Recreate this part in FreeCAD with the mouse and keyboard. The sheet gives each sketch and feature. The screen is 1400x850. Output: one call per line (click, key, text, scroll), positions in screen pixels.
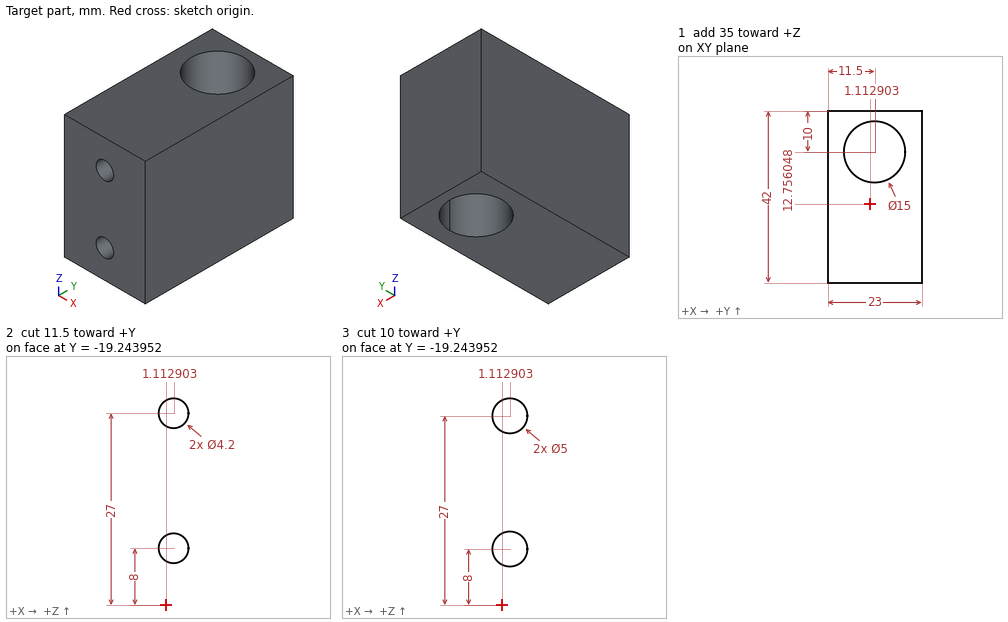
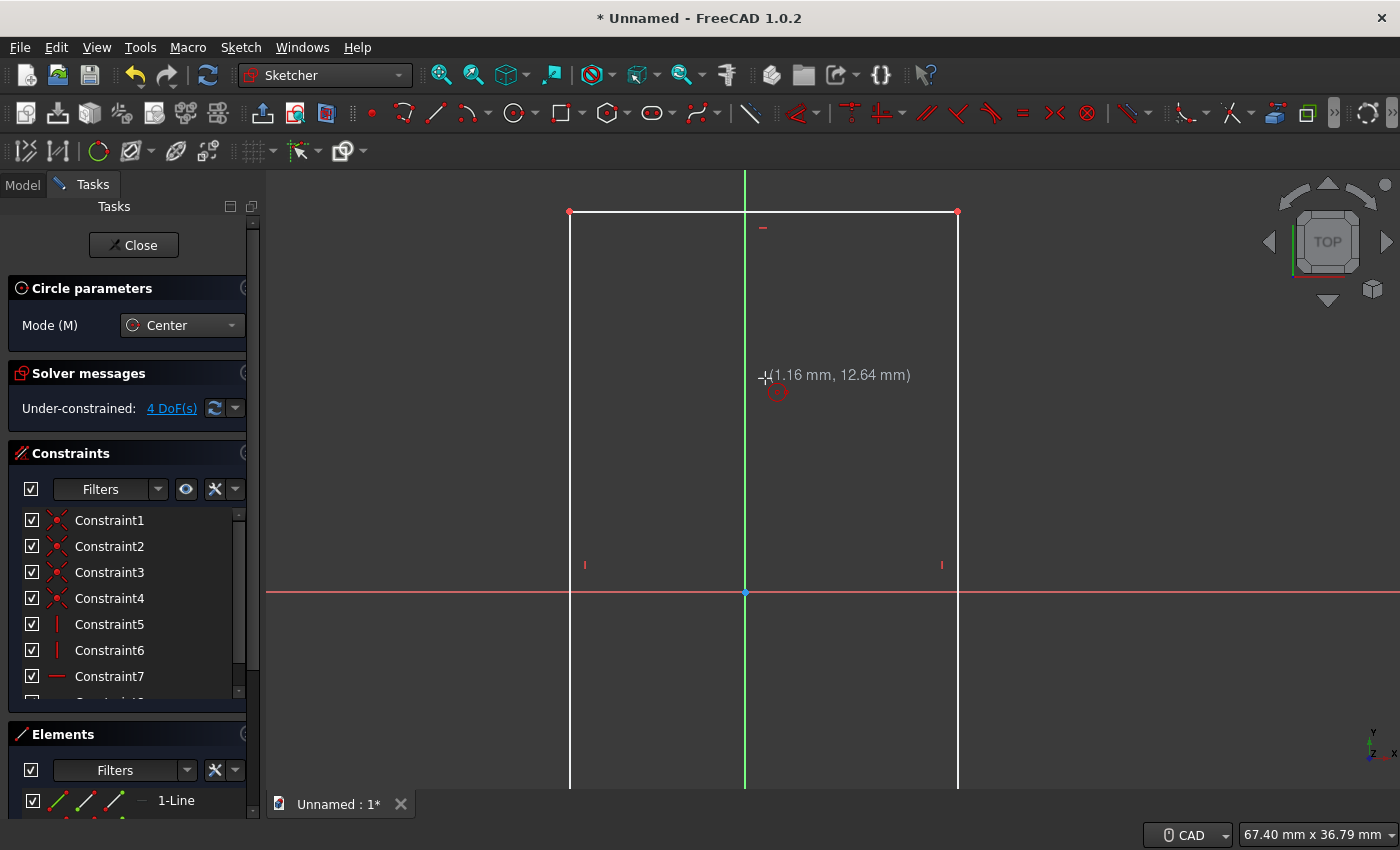
click(764, 378)
click(853, 288)
key(Escape)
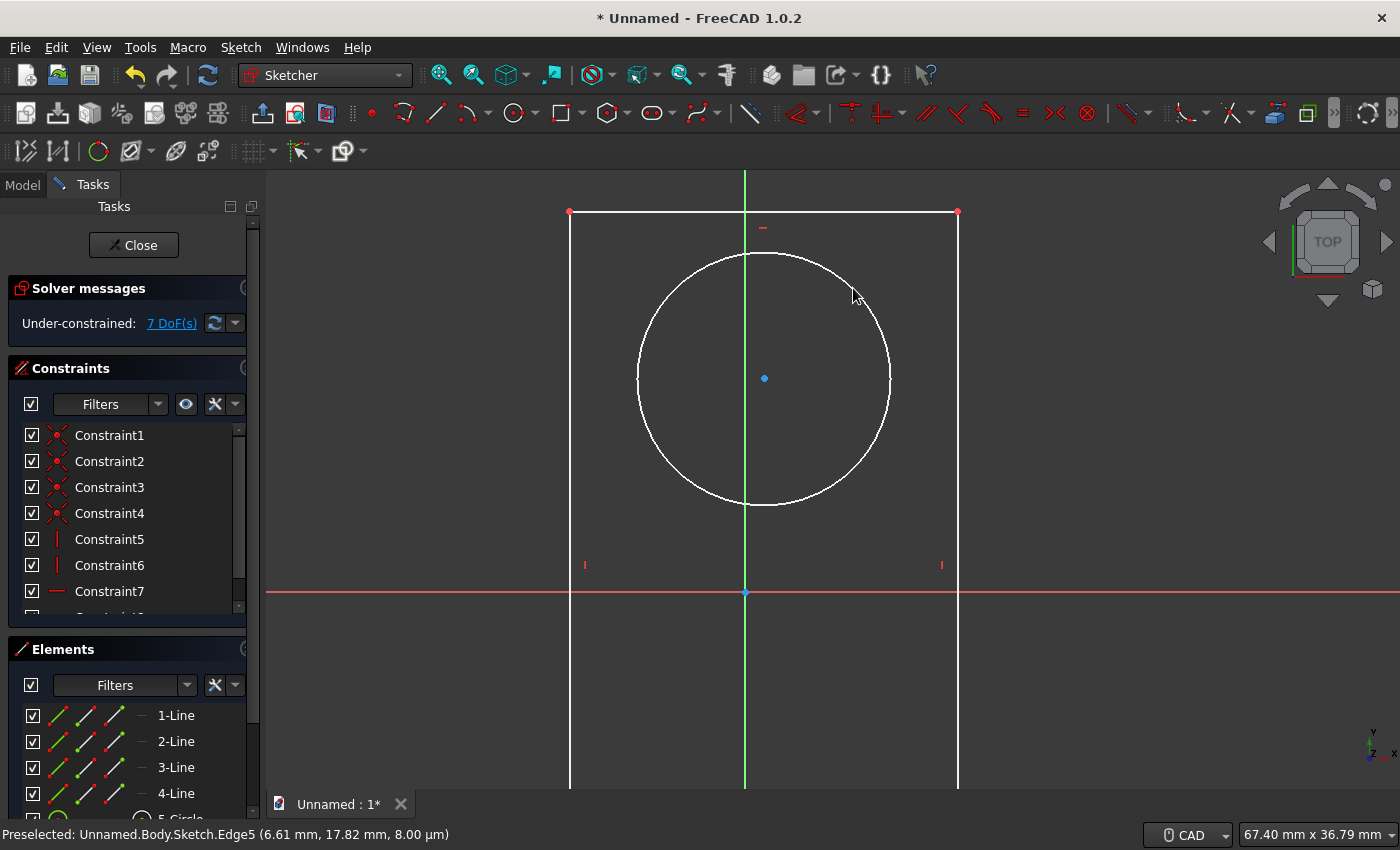
click(796, 114)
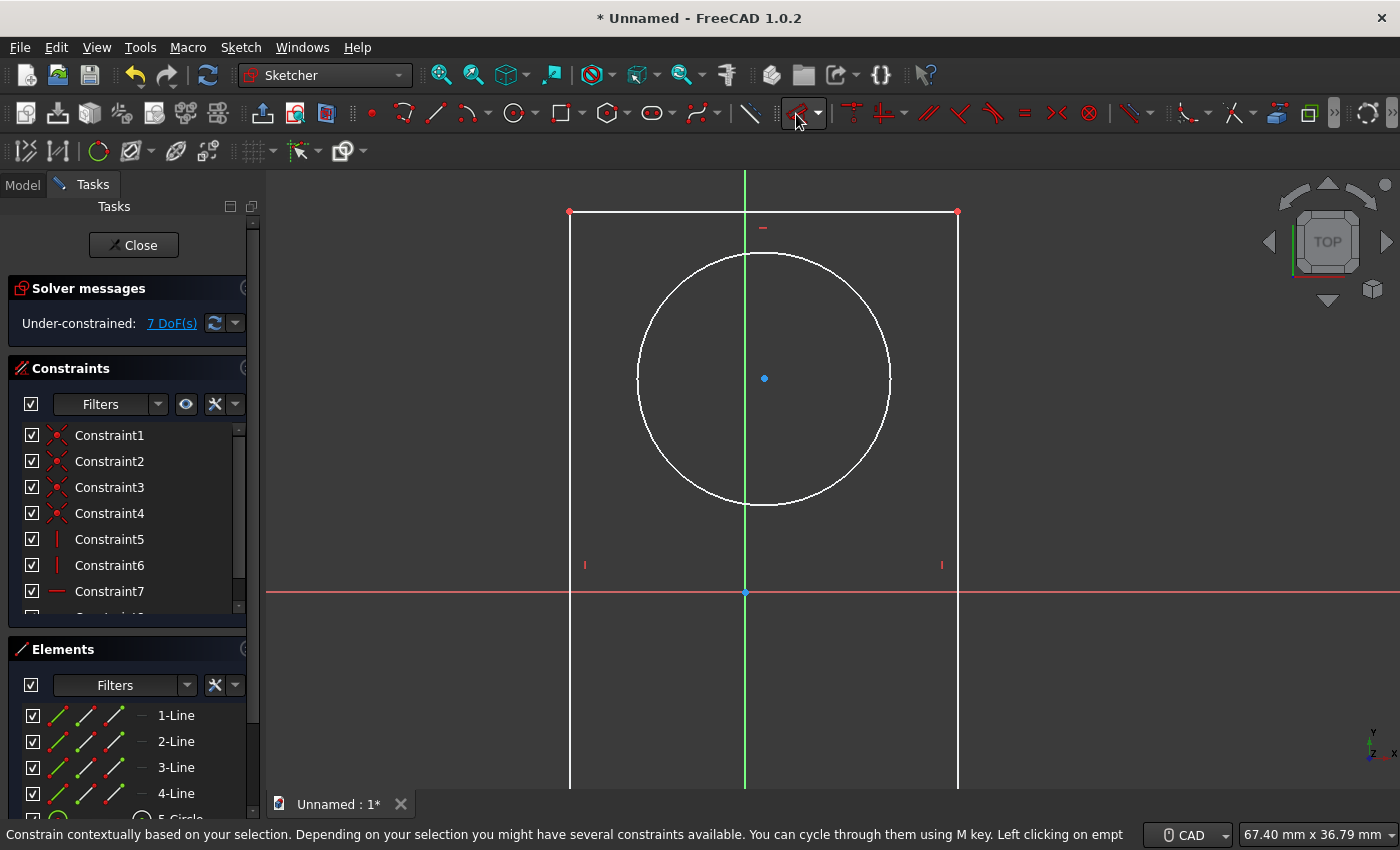
click(853, 289)
click(876, 266)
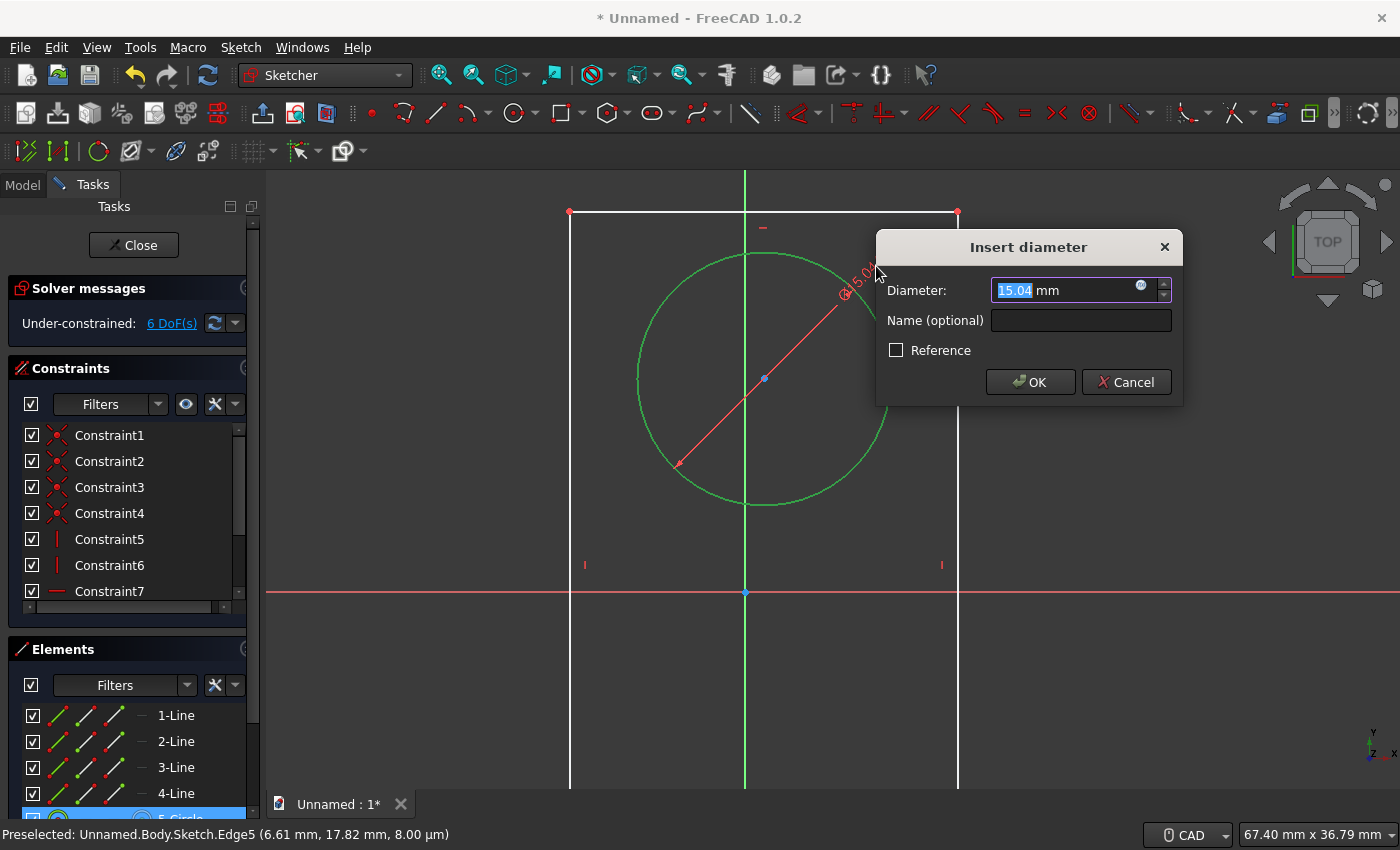
text(15)
key(Return)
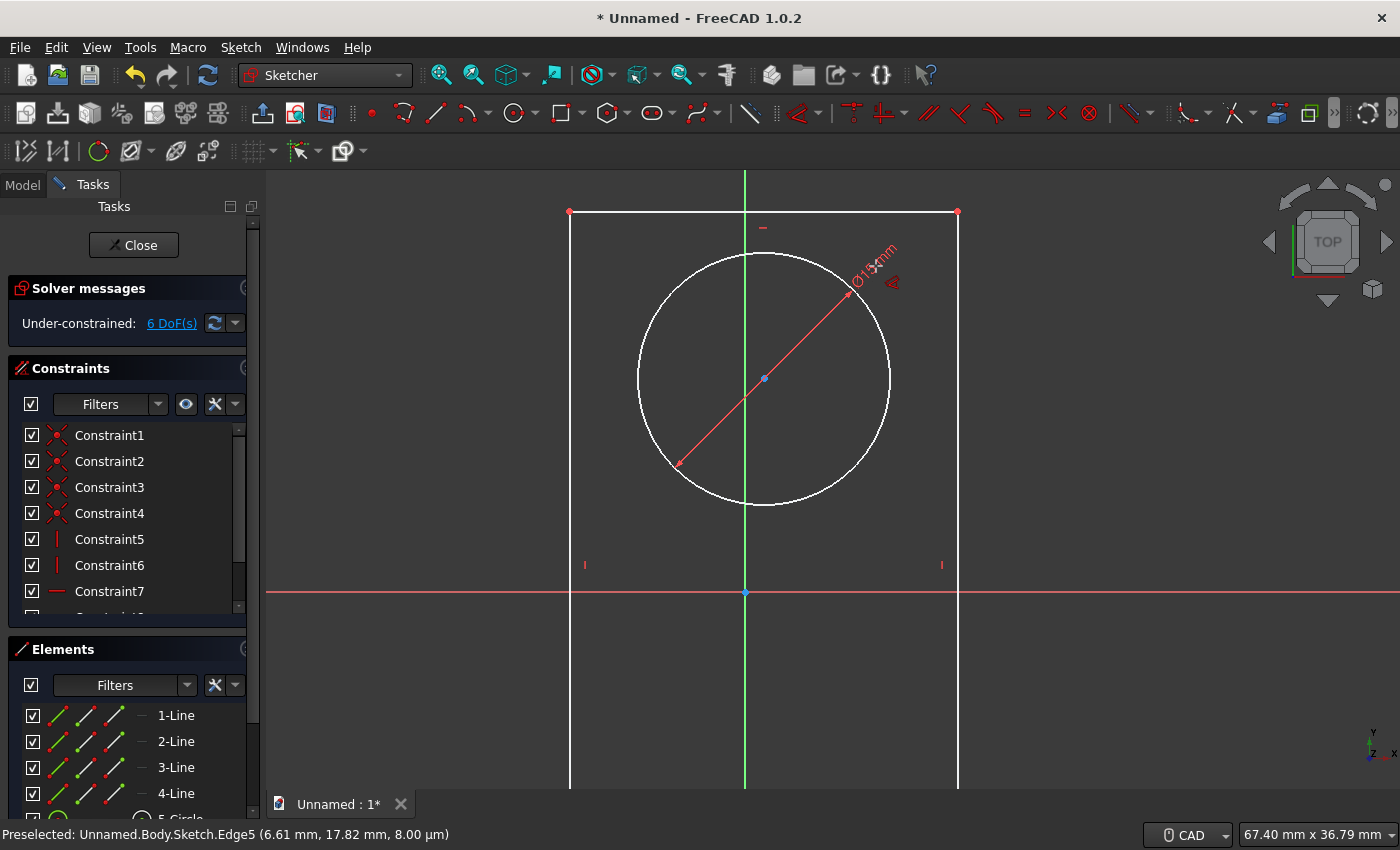
click(570, 423)
click(536, 486)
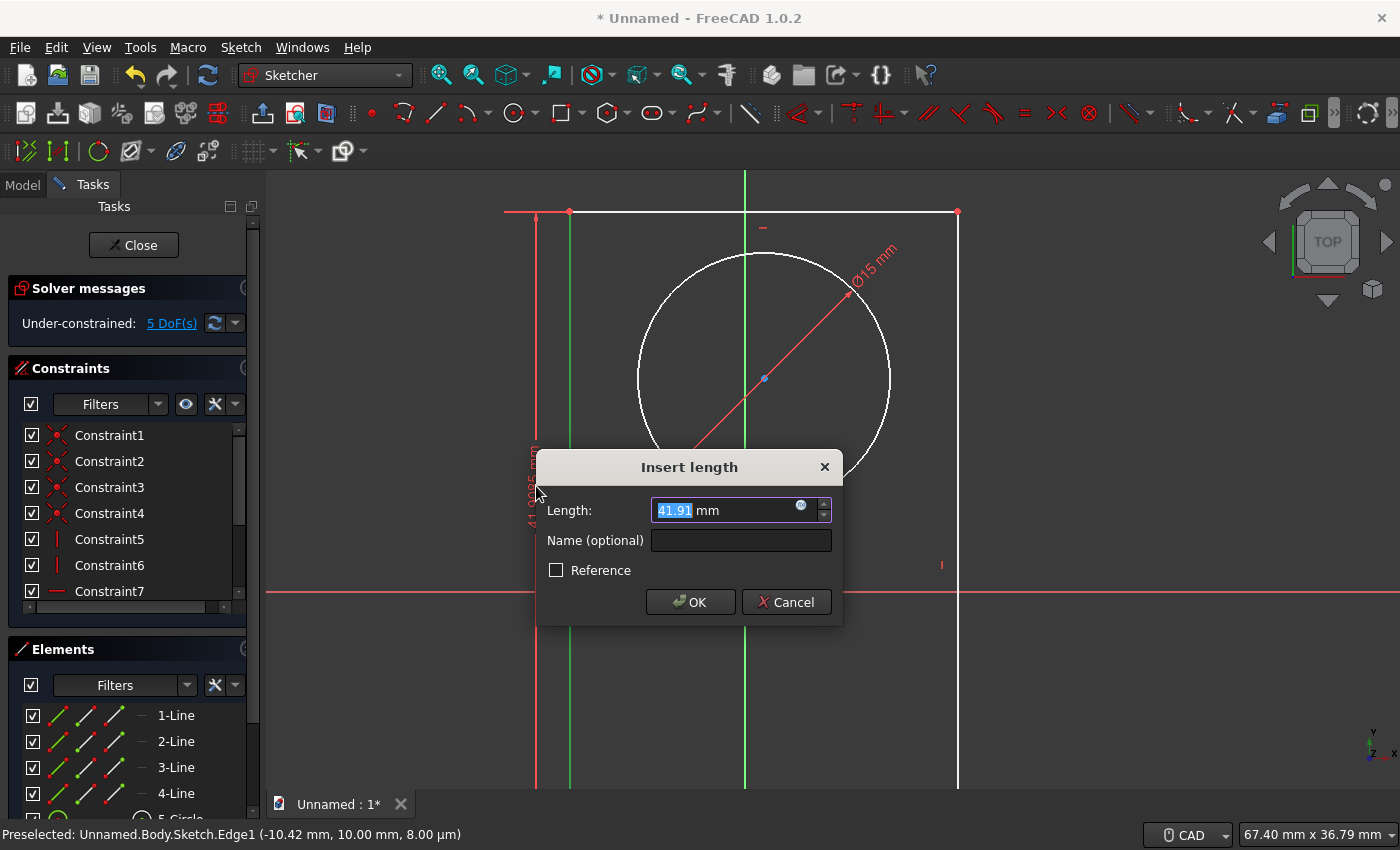
text(42)
key(Return)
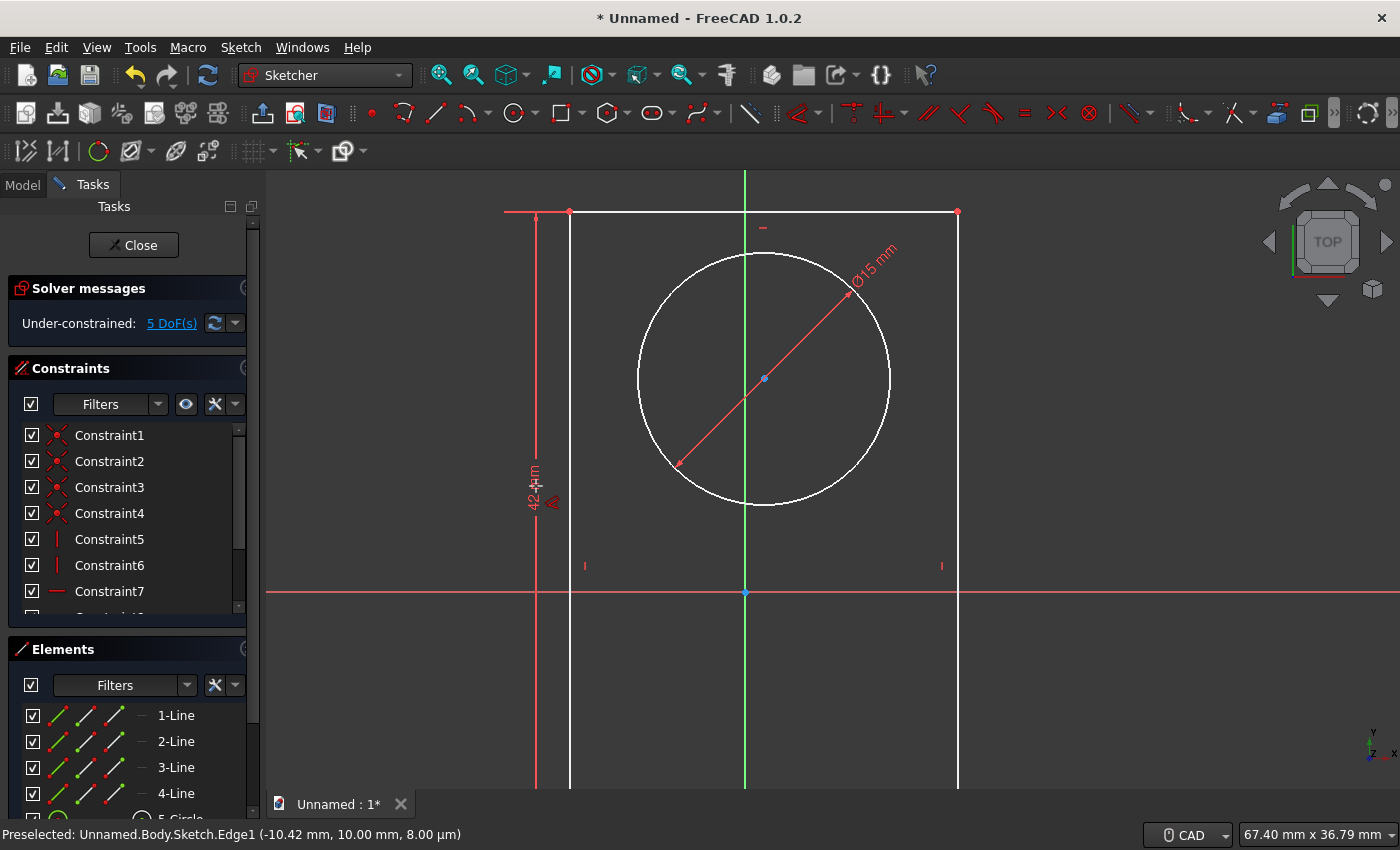
scroll(765, 378, down, 3)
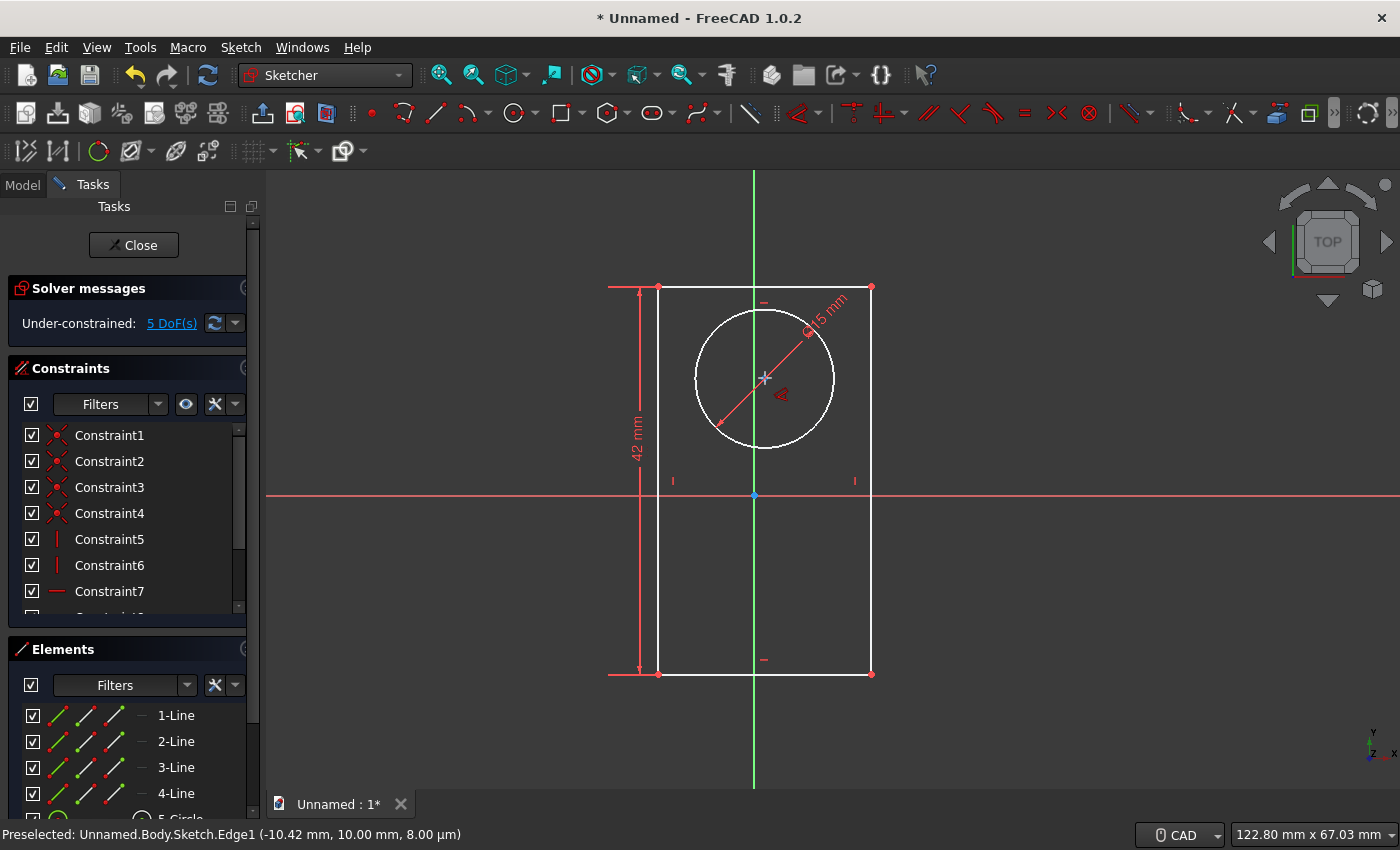
click(722, 675)
click(716, 709)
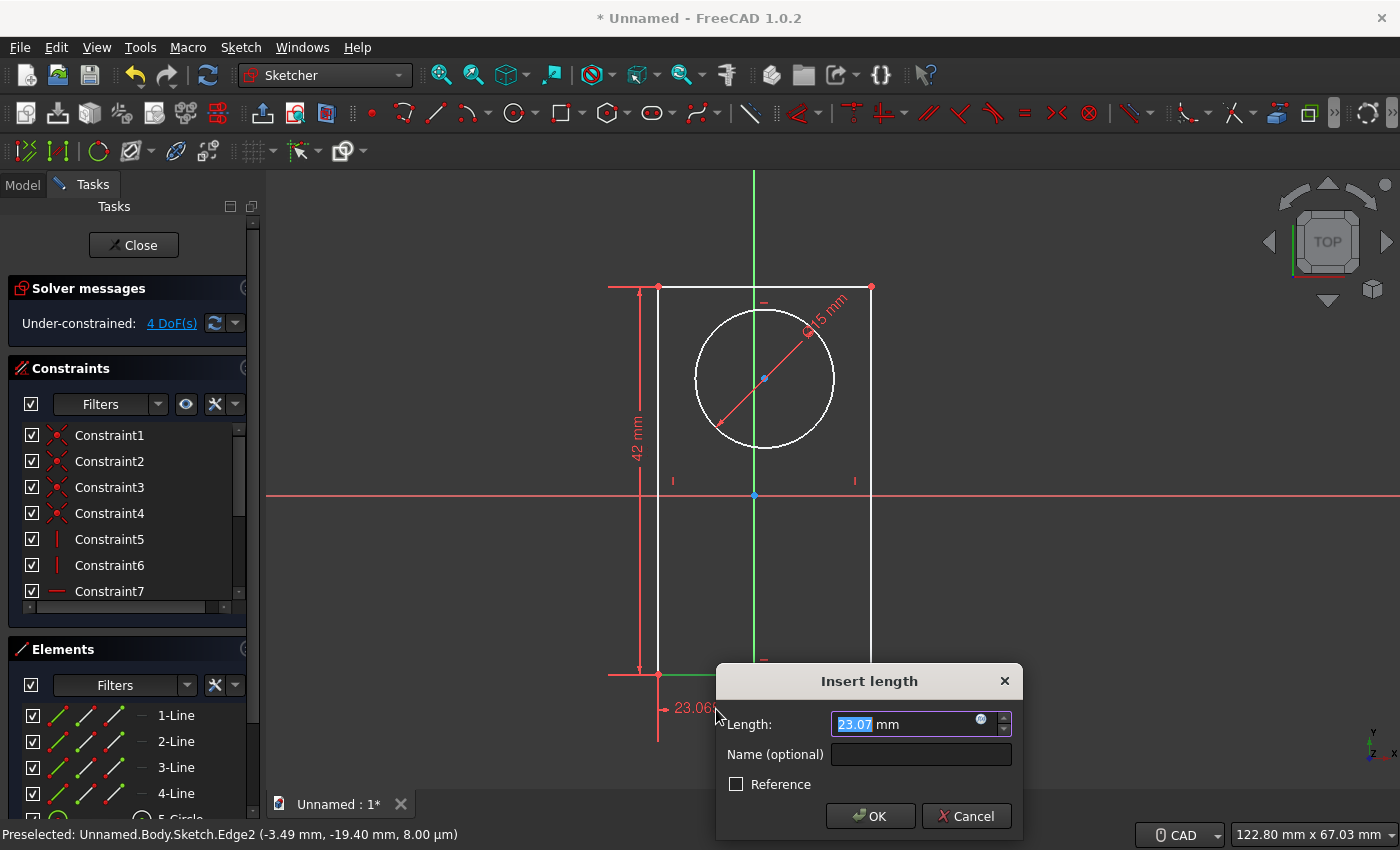
text(23)
key(Return)